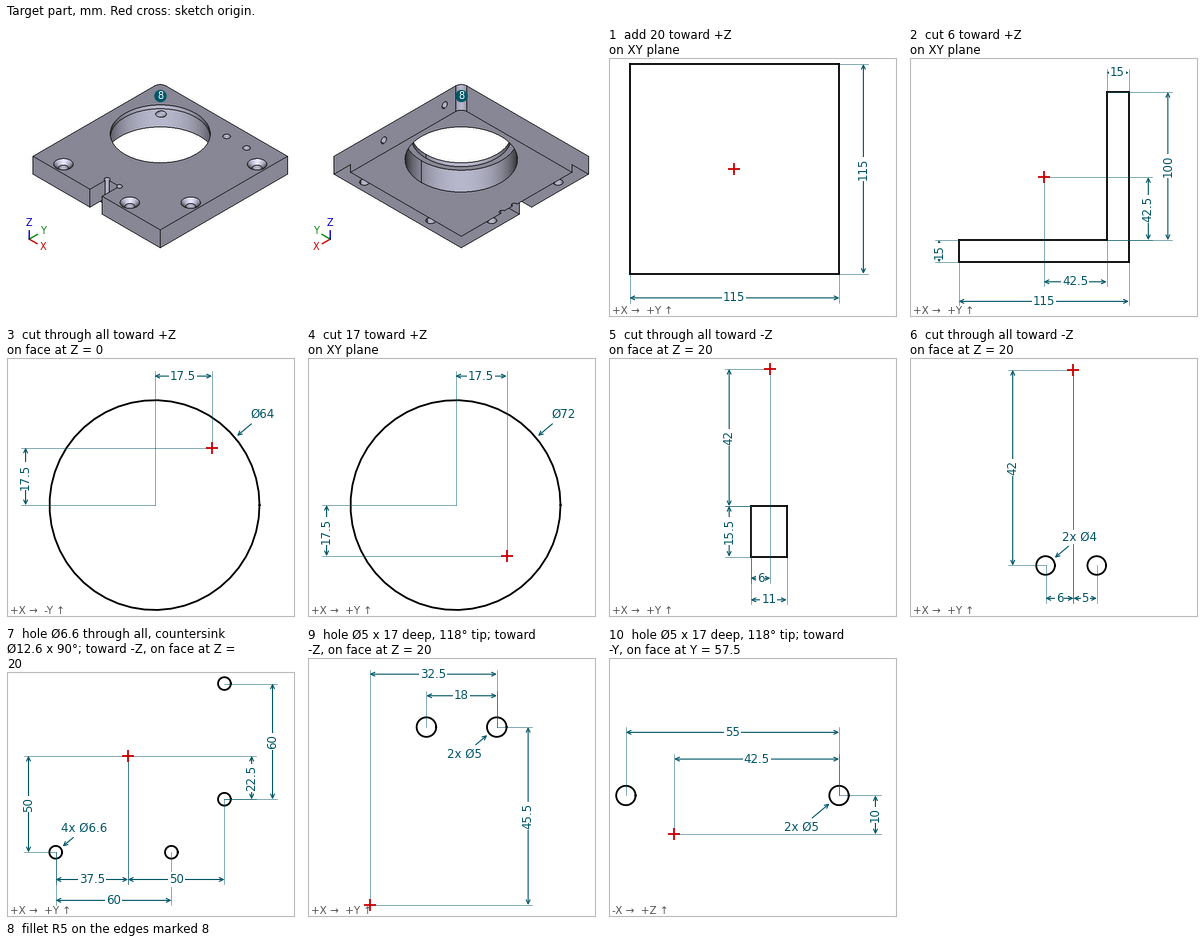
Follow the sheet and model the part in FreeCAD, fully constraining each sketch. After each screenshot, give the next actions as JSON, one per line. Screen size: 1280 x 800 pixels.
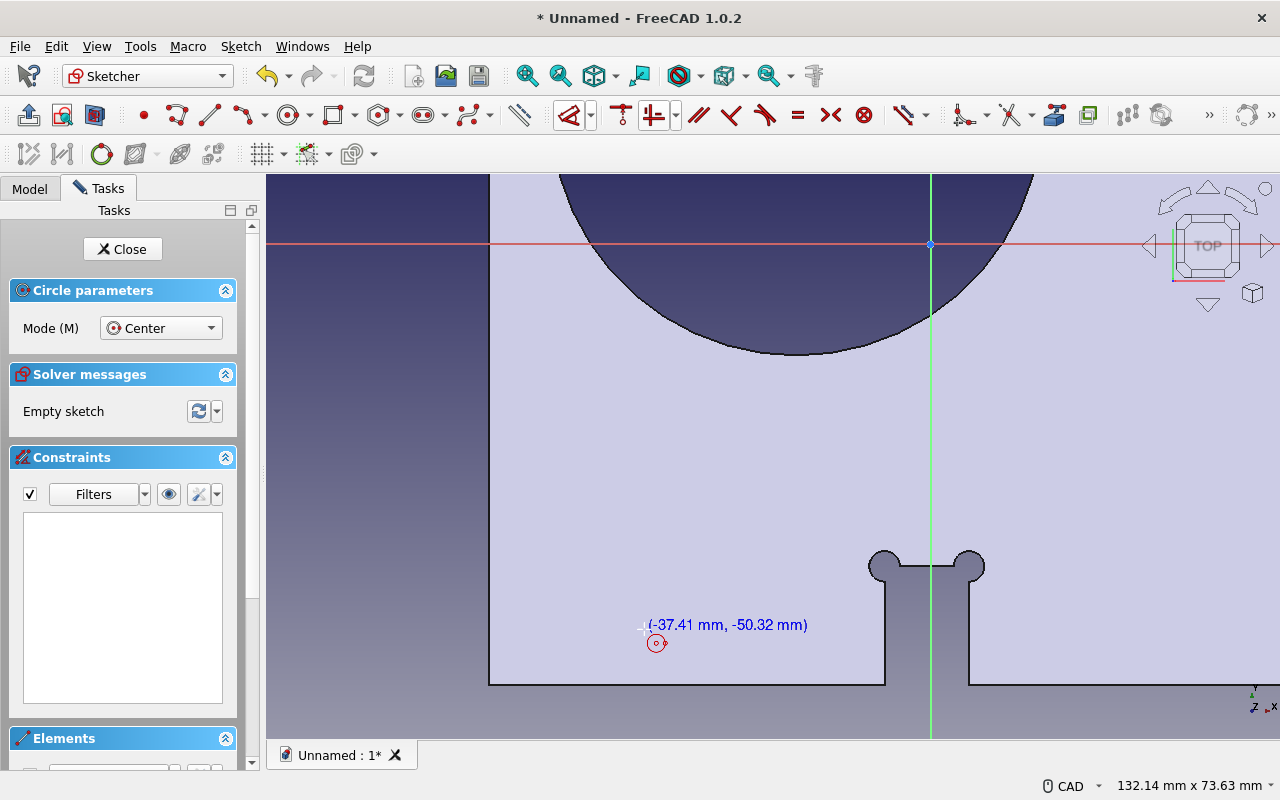
{"action": "left_click", "coordinate": [643, 628]}
{"action": "left_click", "coordinate": [661, 610]}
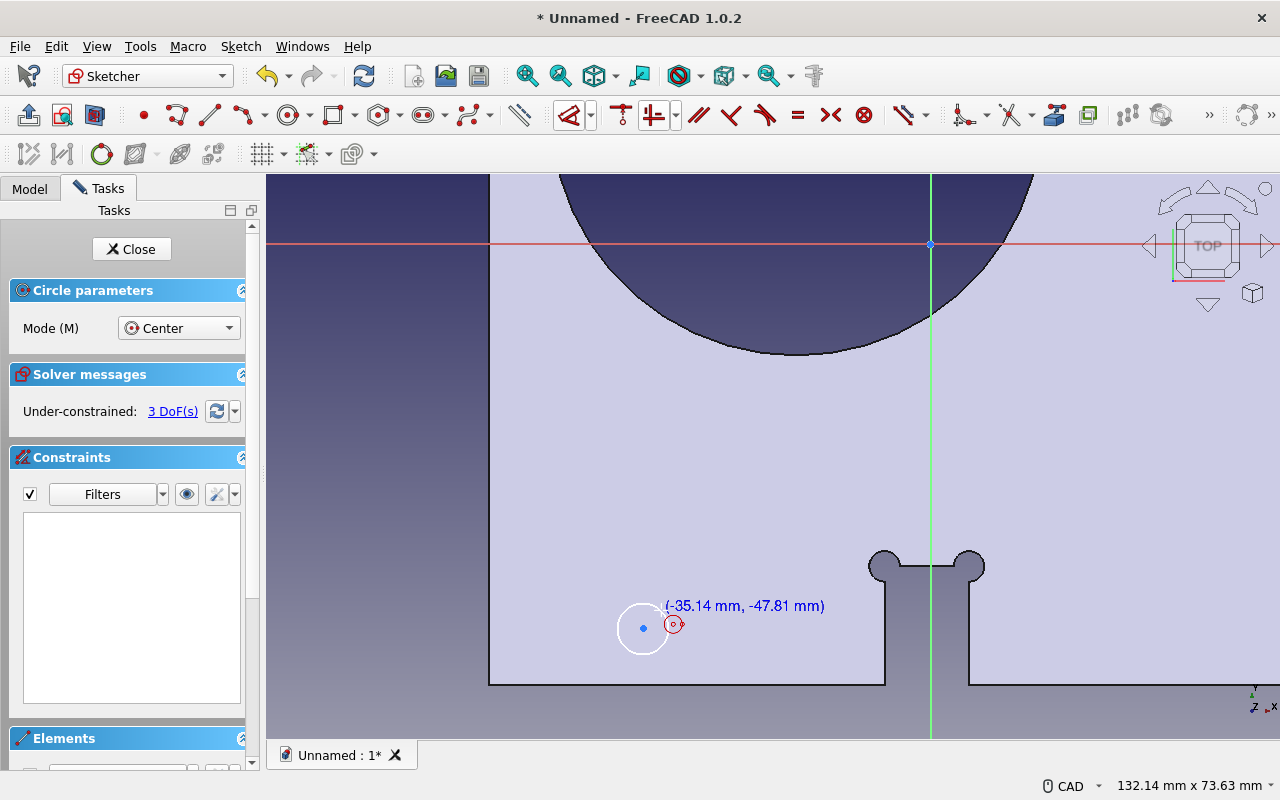
{"action": "left_click", "coordinate": [1103, 628]}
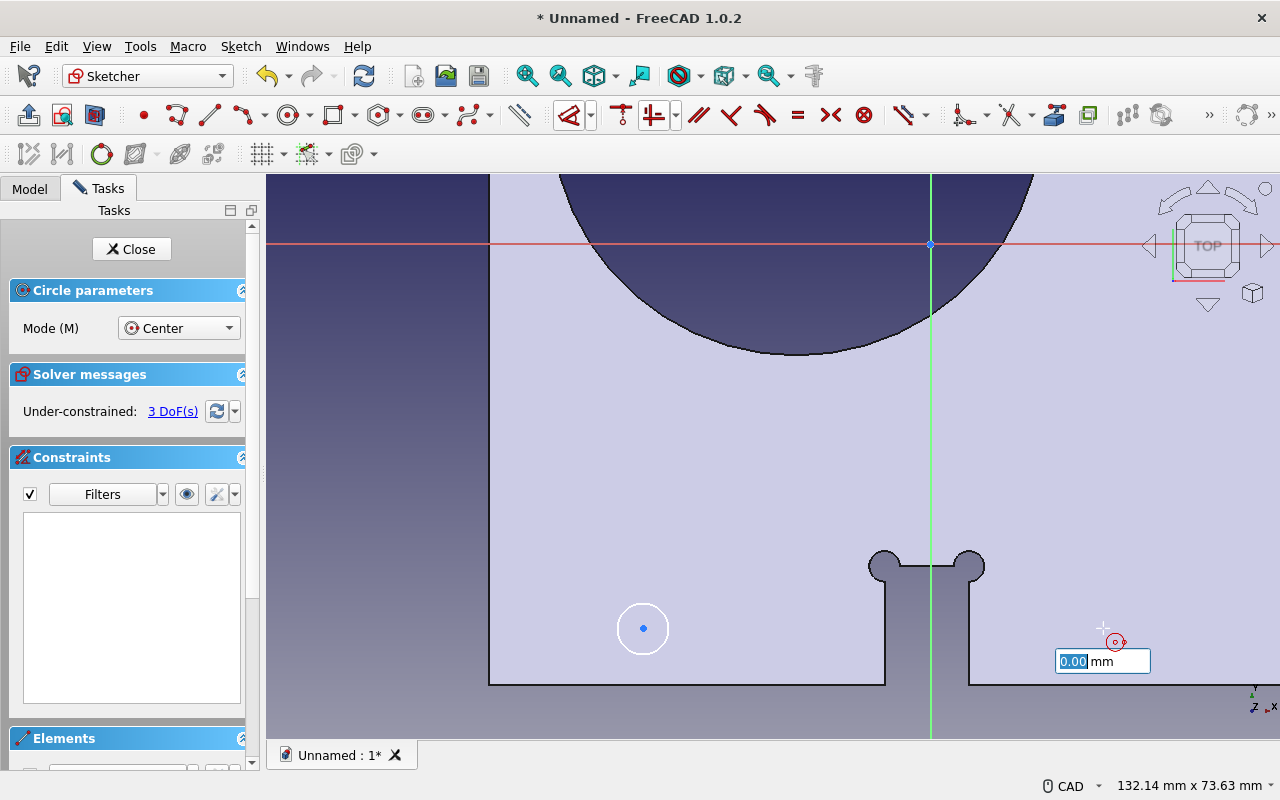
{"action": "scroll", "coordinate": [371, 657], "scroll_direction": "down", "scroll_amount": 3}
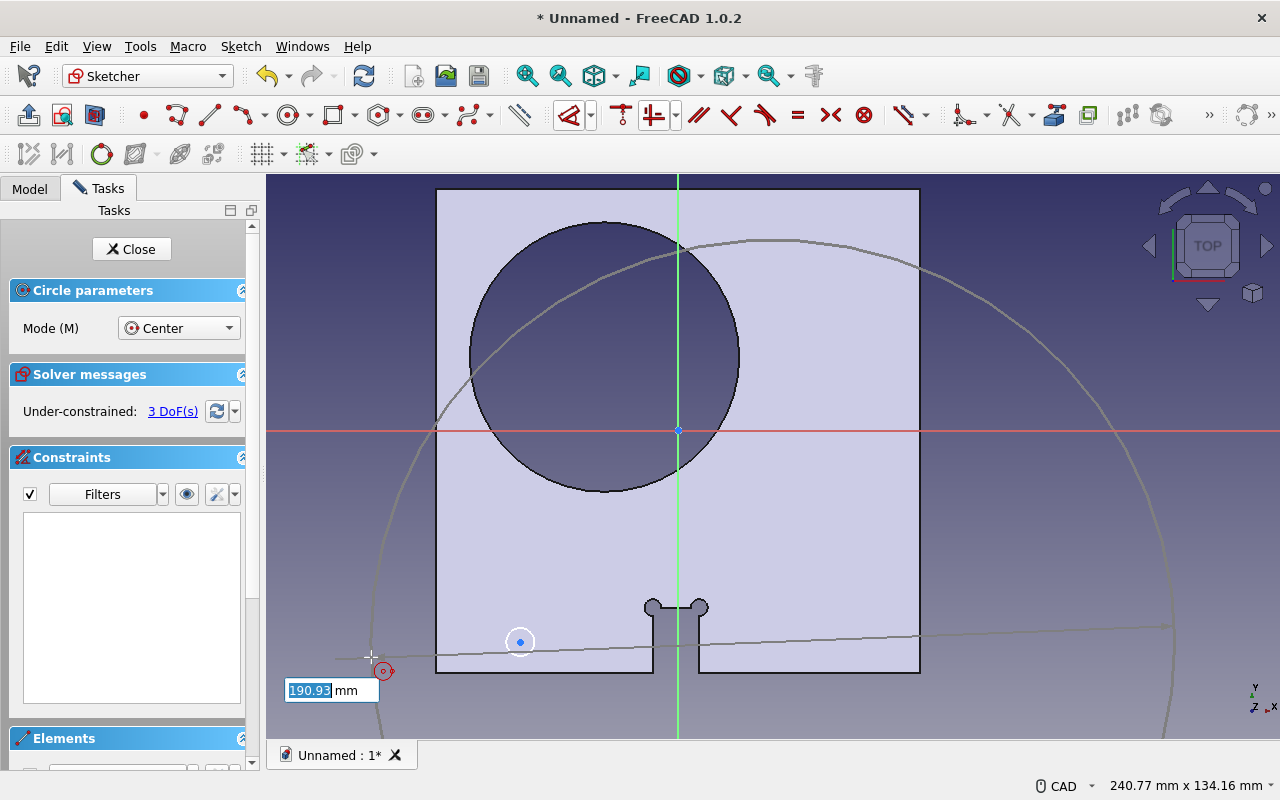
{"action": "left_click", "coordinate": [783, 632]}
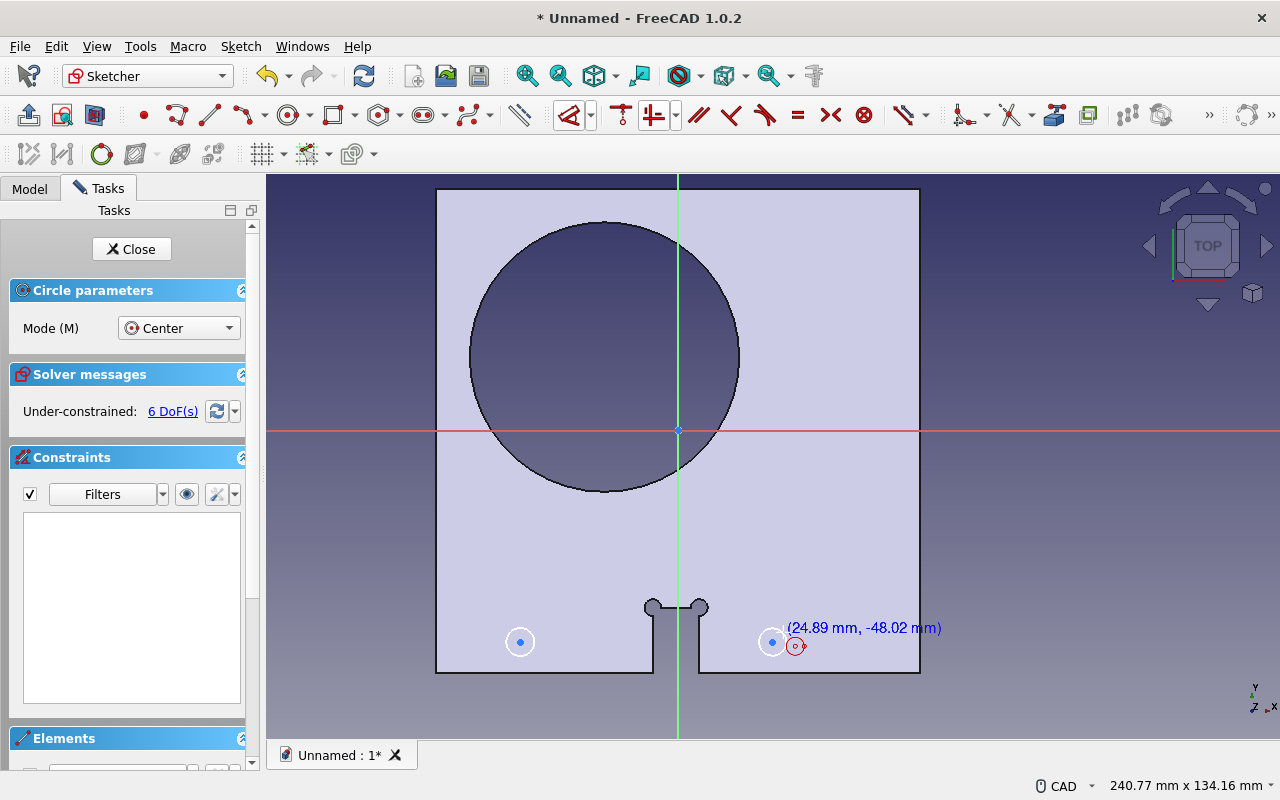
{"action": "scroll", "coordinate": [889, 526], "scroll_direction": "up", "scroll_amount": 3}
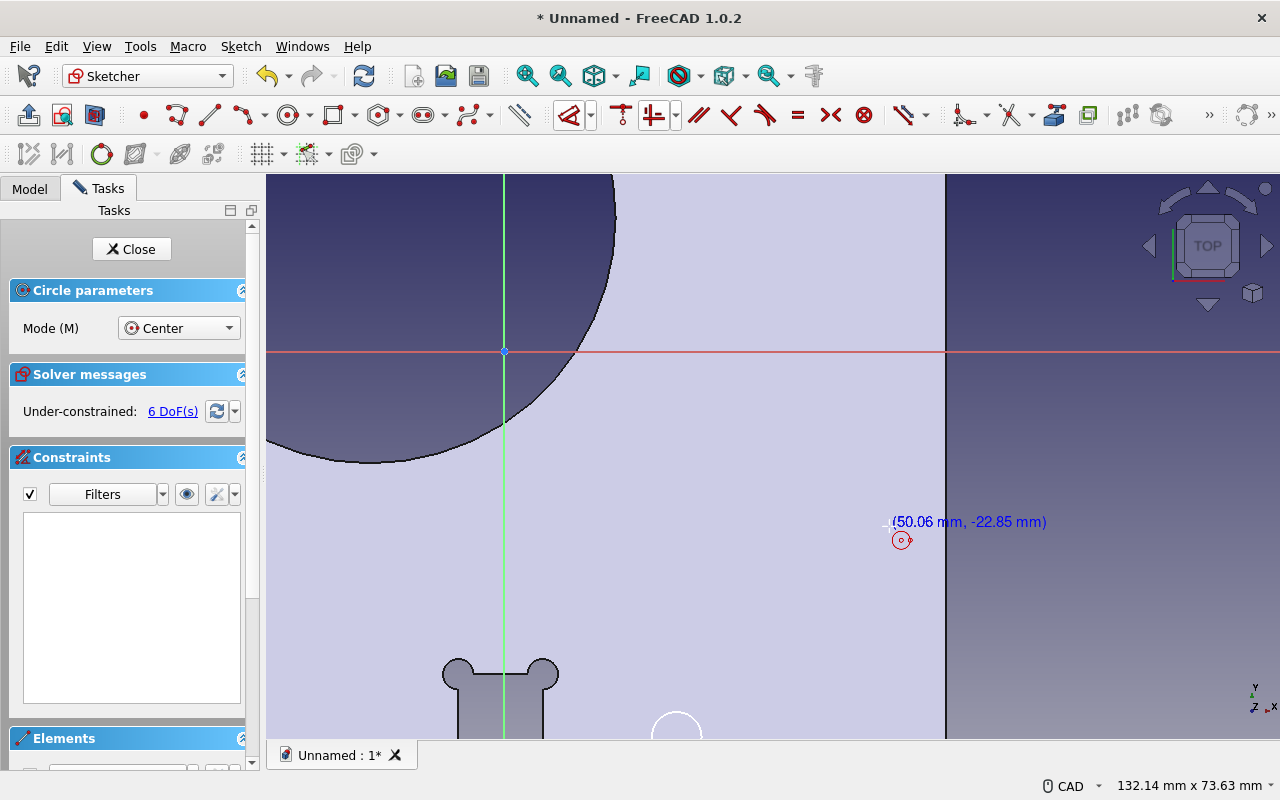
{"action": "left_click", "coordinate": [888, 525]}
{"action": "left_click", "coordinate": [906, 507]}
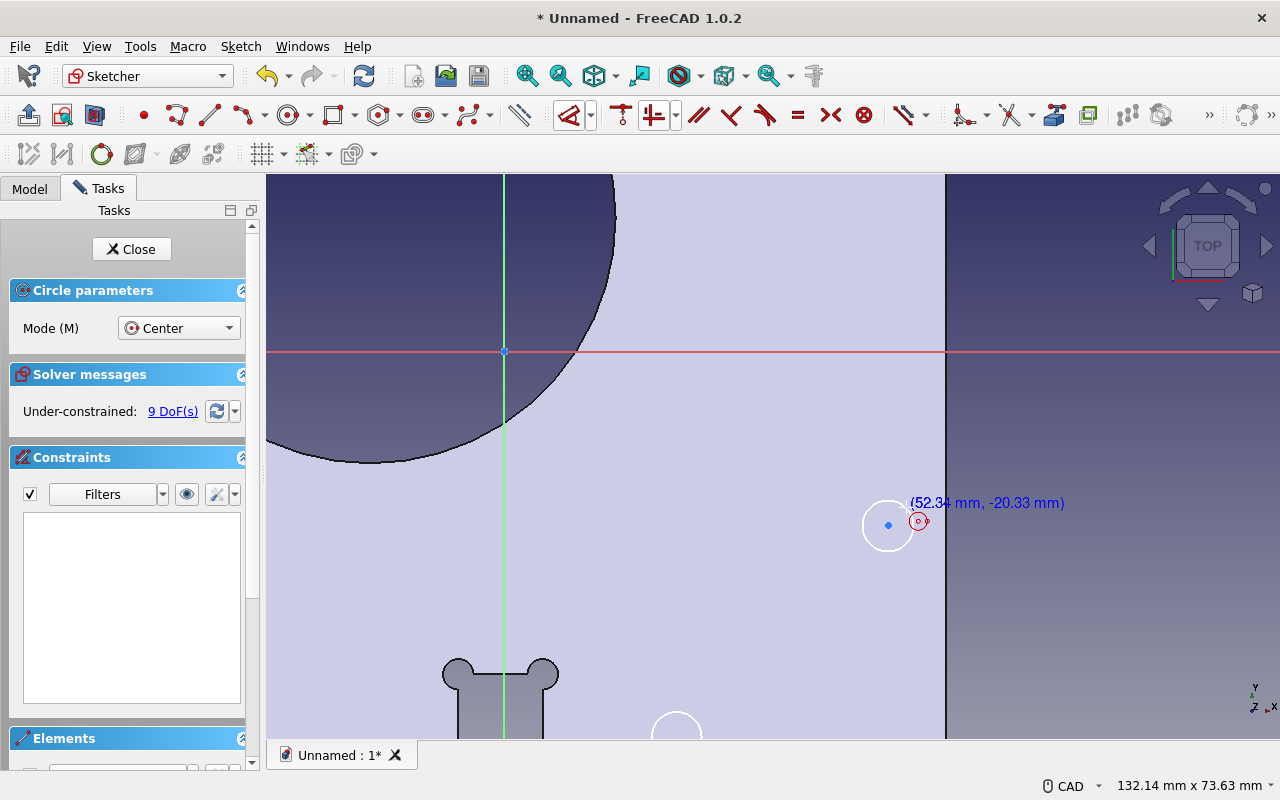
{"action": "scroll", "coordinate": [890, 525], "scroll_direction": "down", "scroll_amount": 3}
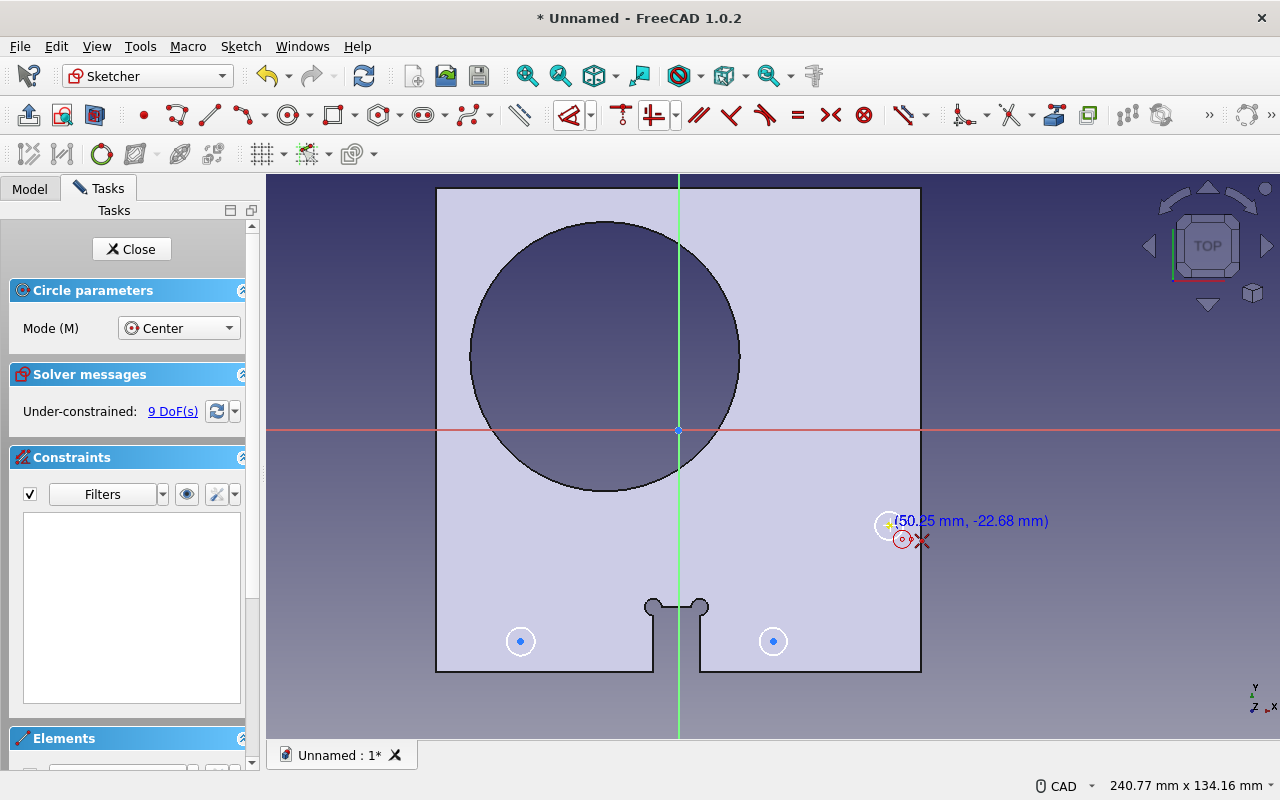
{"action": "scroll", "coordinate": [889, 272], "scroll_direction": "up", "scroll_amount": 3}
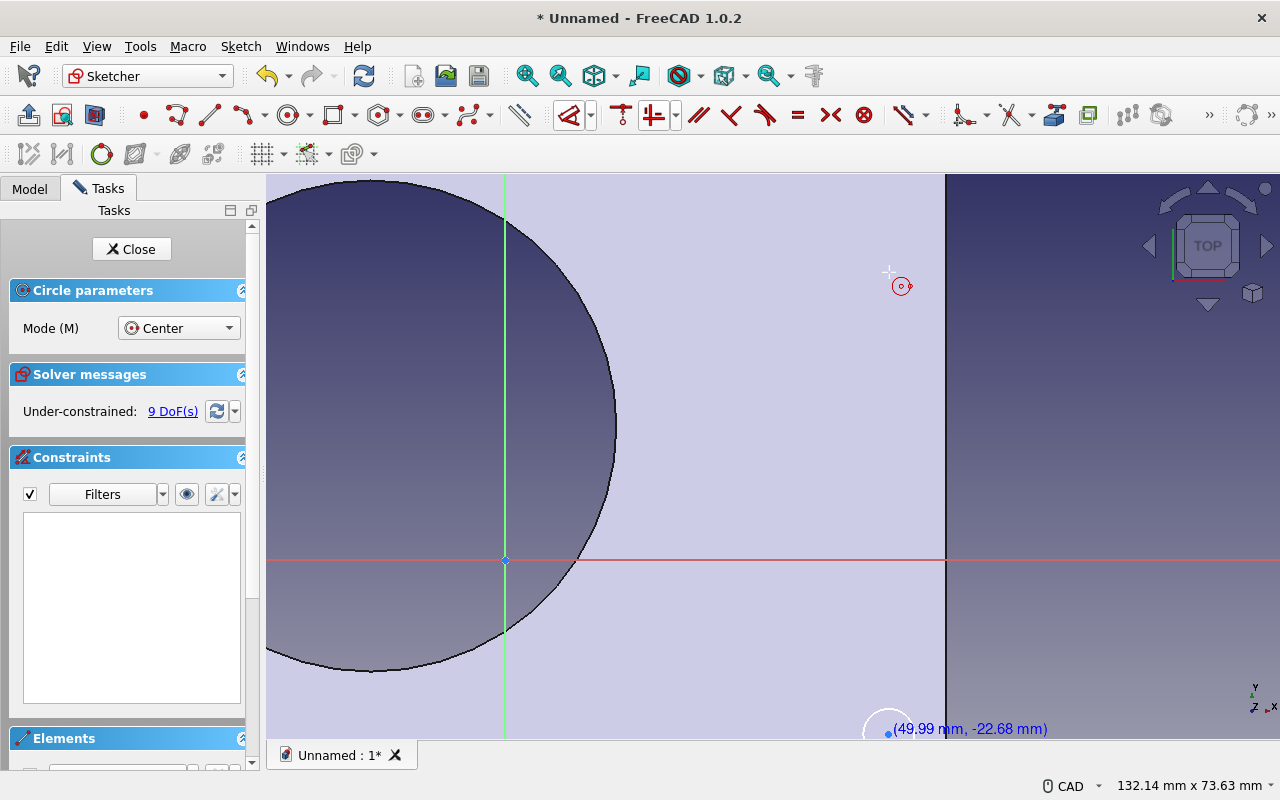
{"action": "left_click", "coordinate": [889, 273]}
{"action": "left_click", "coordinate": [907, 255]}
{"action": "key", "text": "Escape"}